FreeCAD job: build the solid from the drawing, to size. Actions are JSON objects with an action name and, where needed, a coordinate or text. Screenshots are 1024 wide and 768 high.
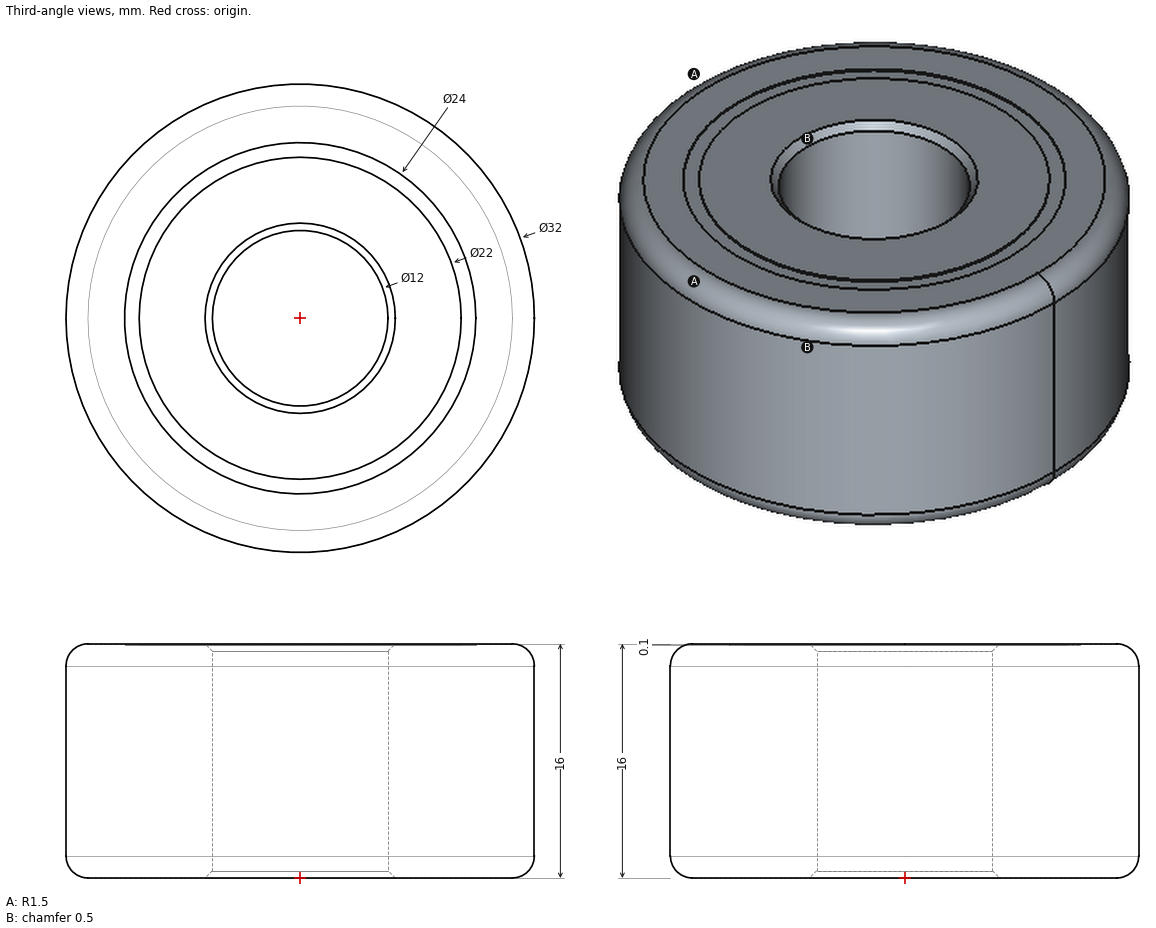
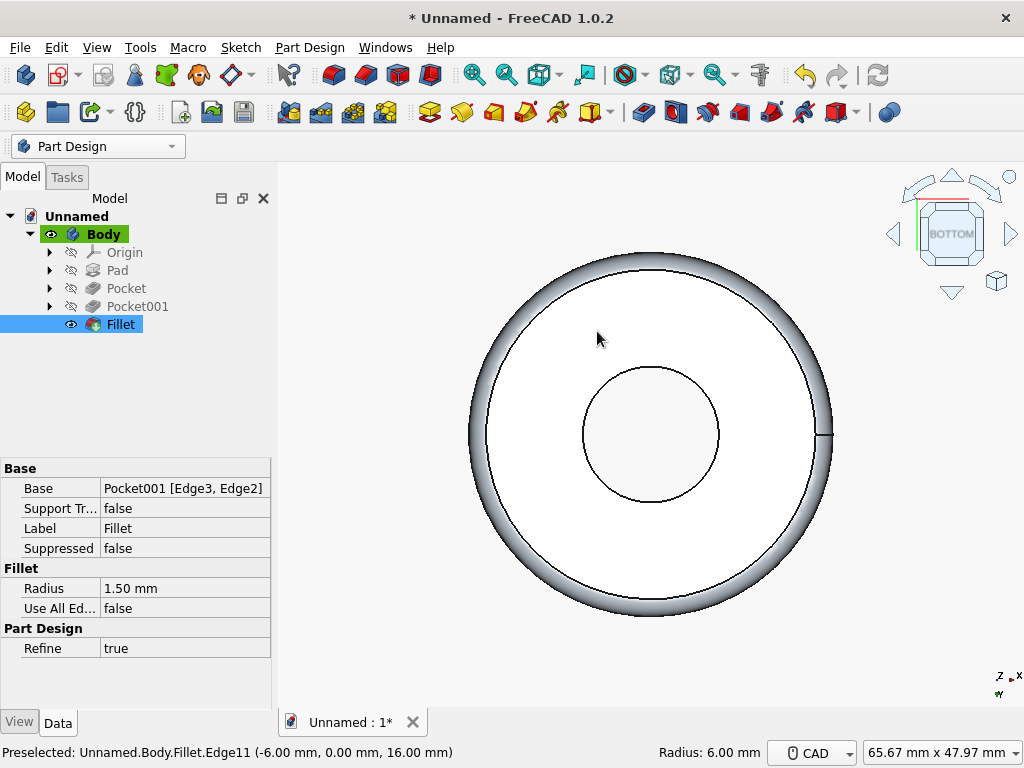
{"action": "left_click", "coordinate": [596, 474], "text": "ctrl"}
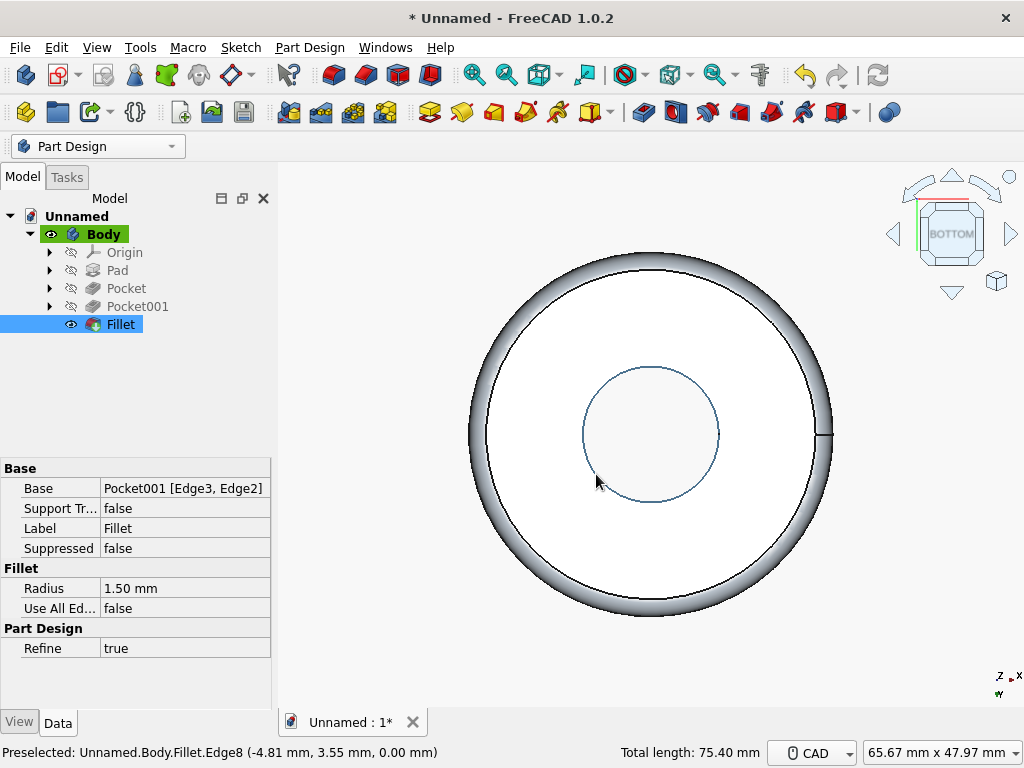
{"action": "left_click", "coordinate": [366, 76]}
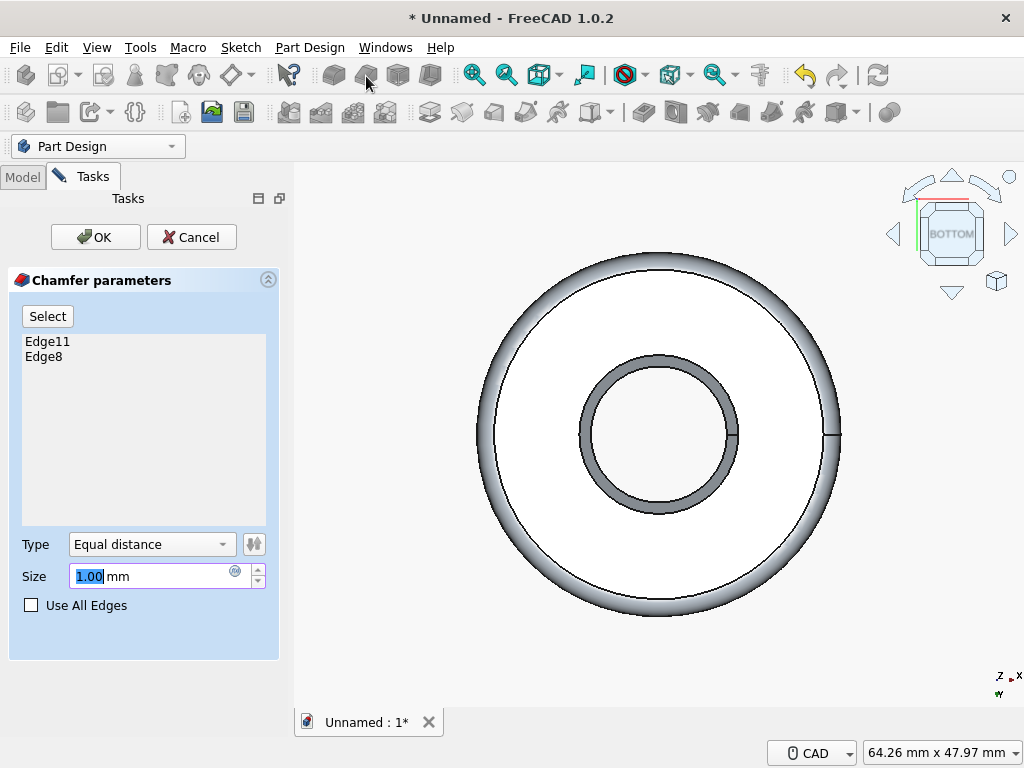
{"action": "type", "text": "0.5"}
{"action": "key", "text": "Tab"}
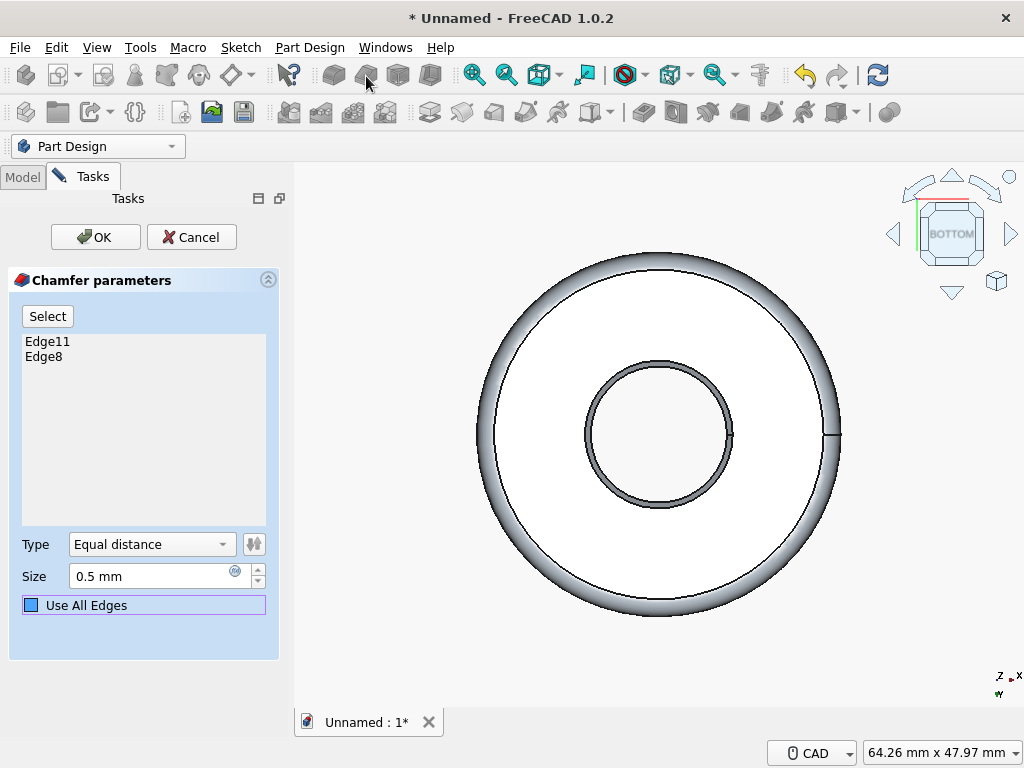
{"action": "left_click", "coordinate": [96, 237]}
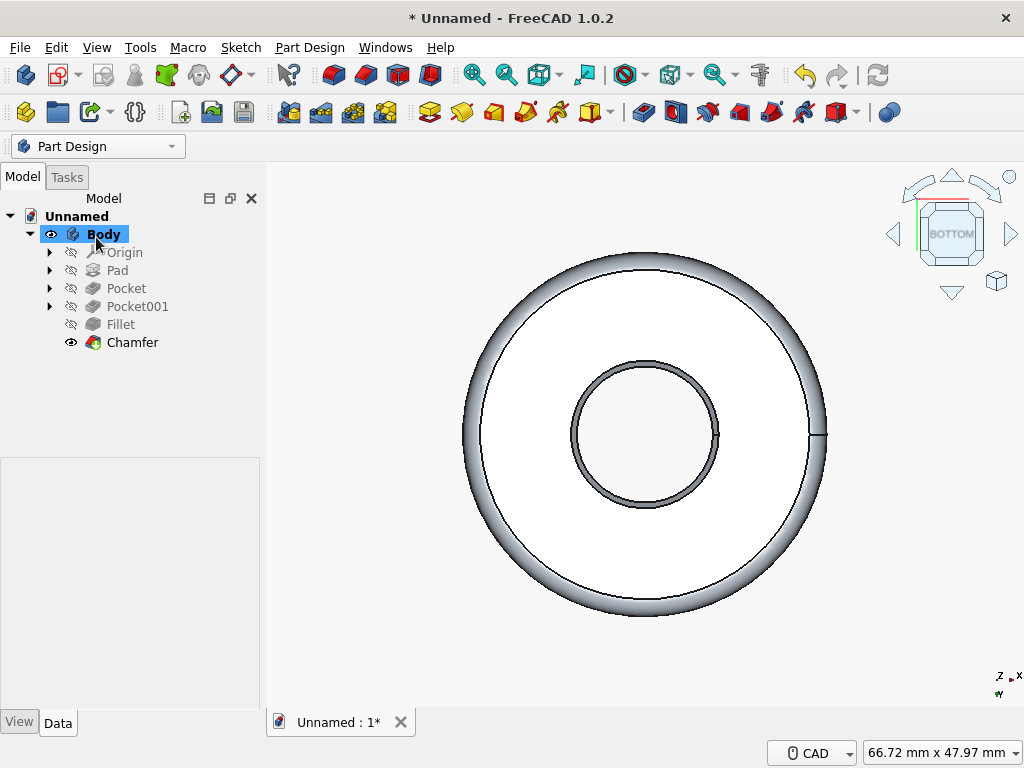
{"action": "key", "text": "0"}